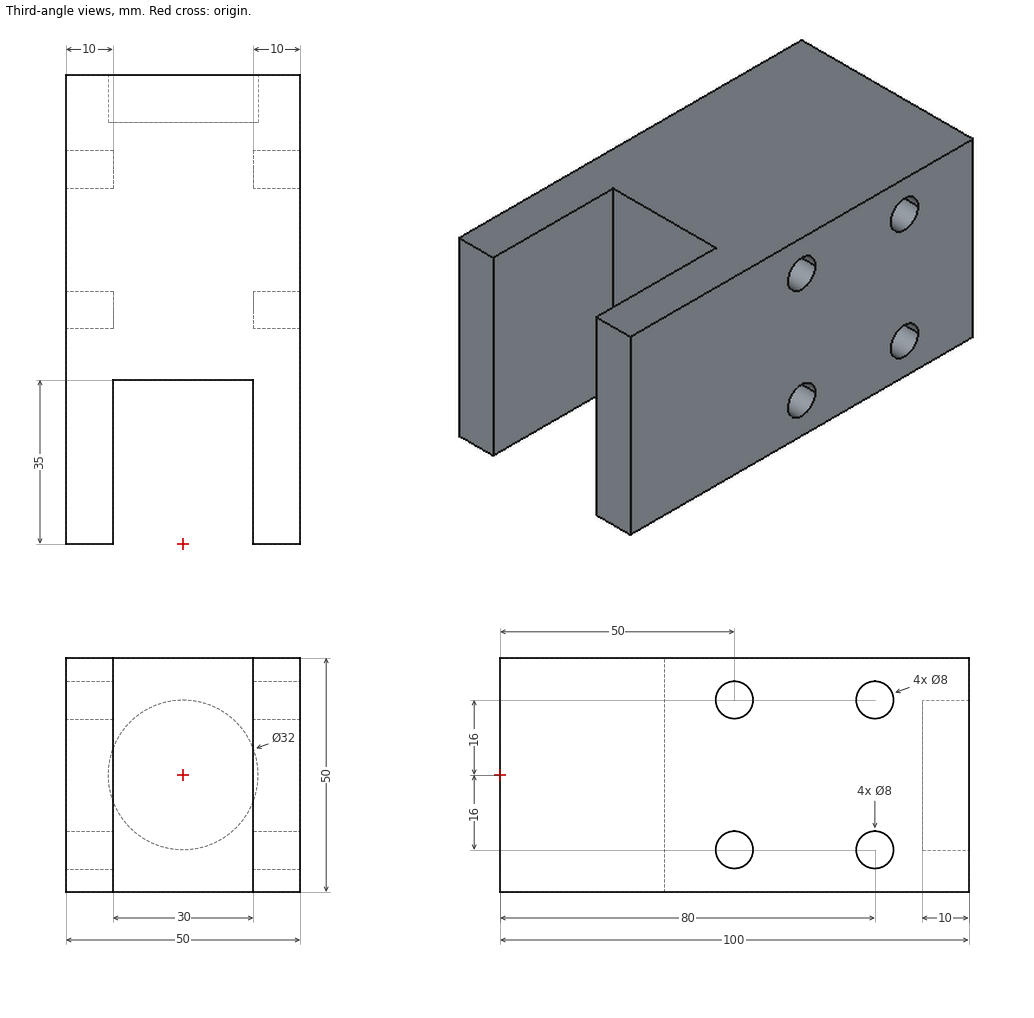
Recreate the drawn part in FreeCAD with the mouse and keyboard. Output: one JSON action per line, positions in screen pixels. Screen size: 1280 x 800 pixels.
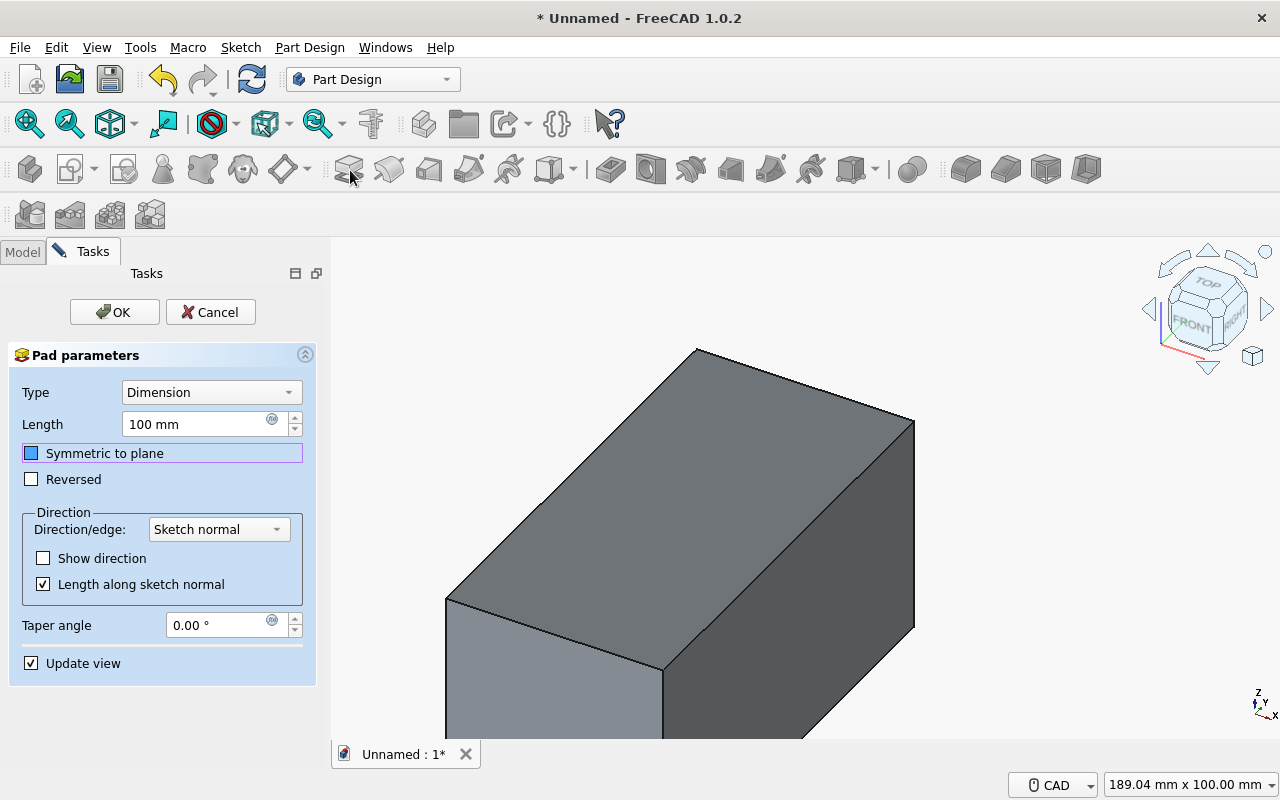
{"action": "left_click", "coordinate": [30, 479]}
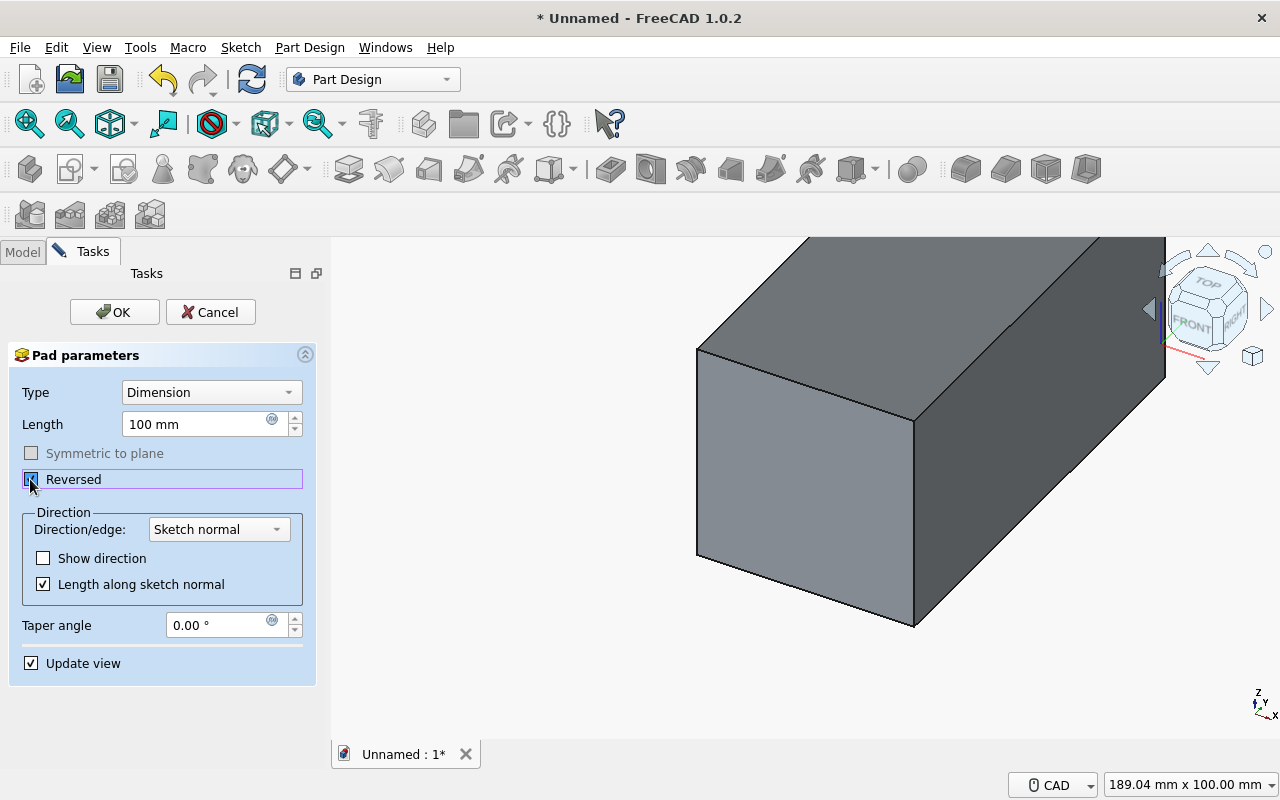
{"action": "left_click", "coordinate": [115, 312]}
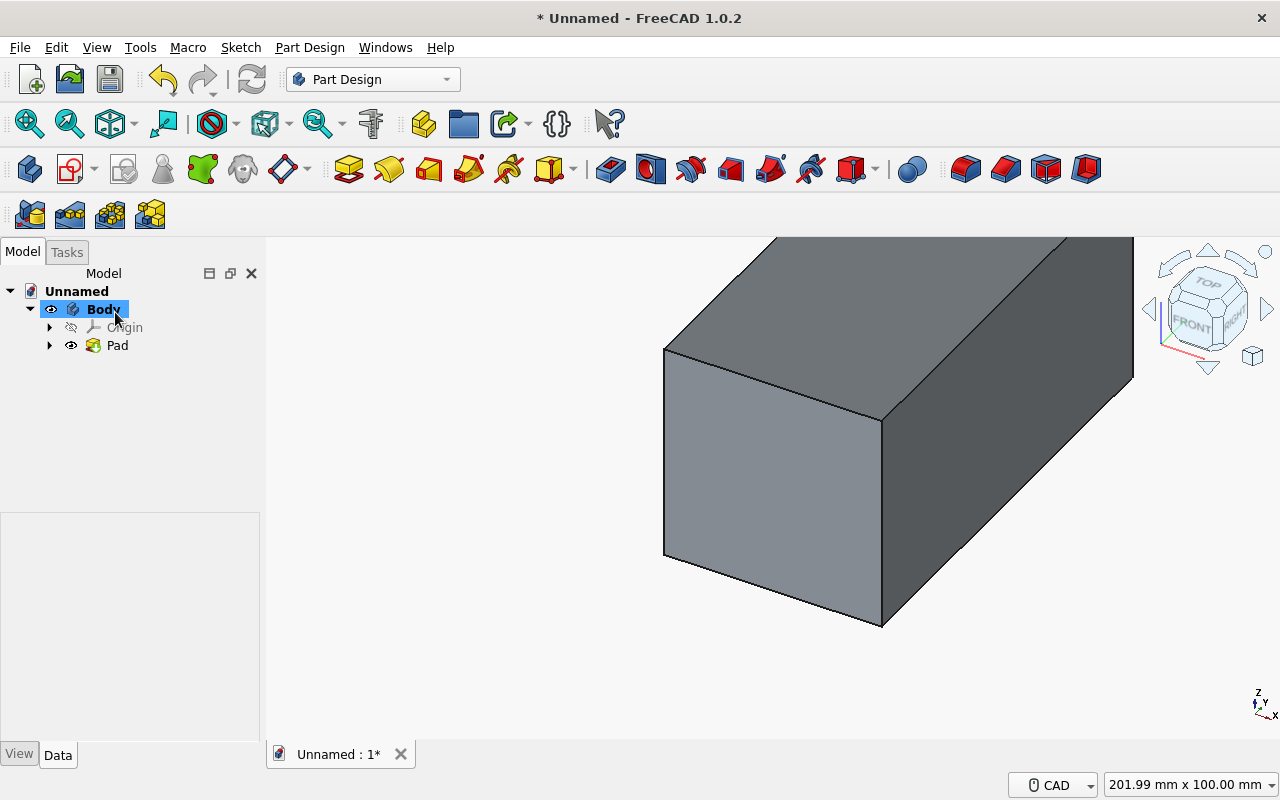
{"action": "left_click", "coordinate": [30, 124]}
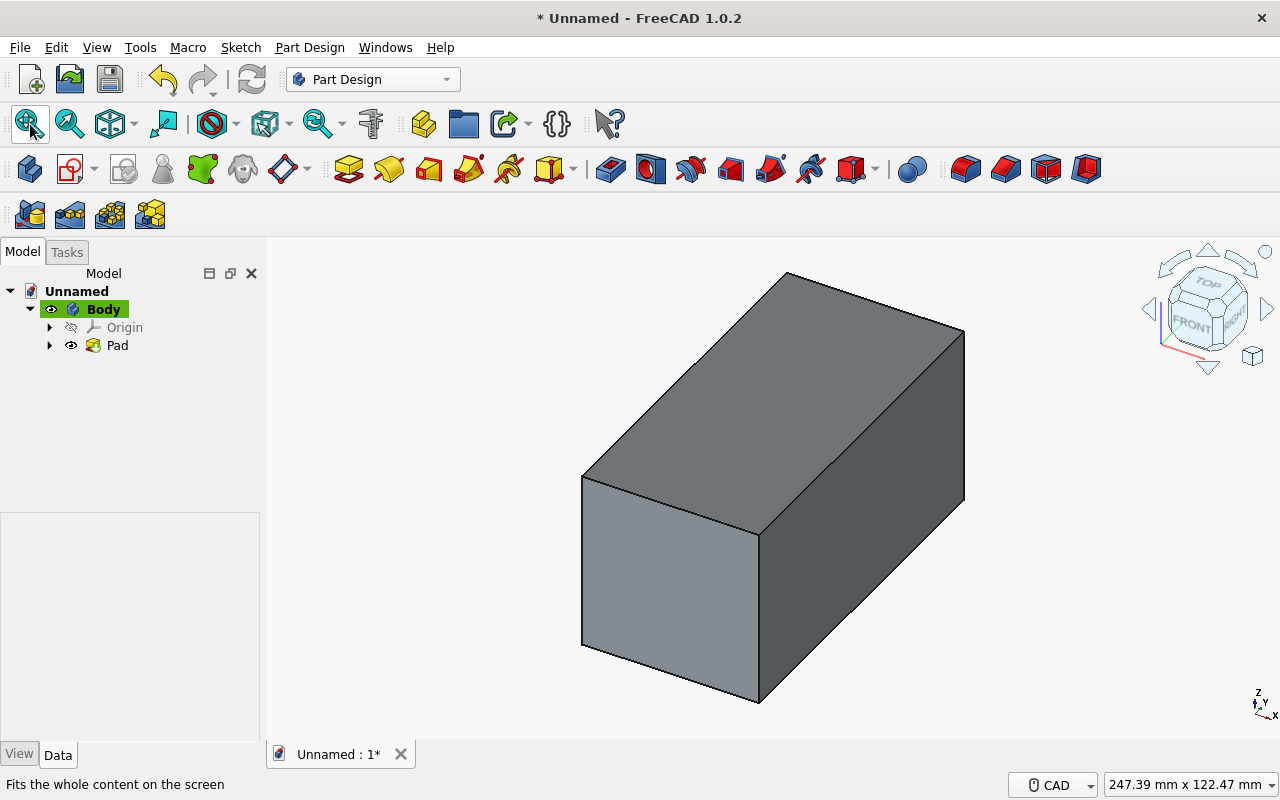
{"action": "left_click", "coordinate": [671, 589]}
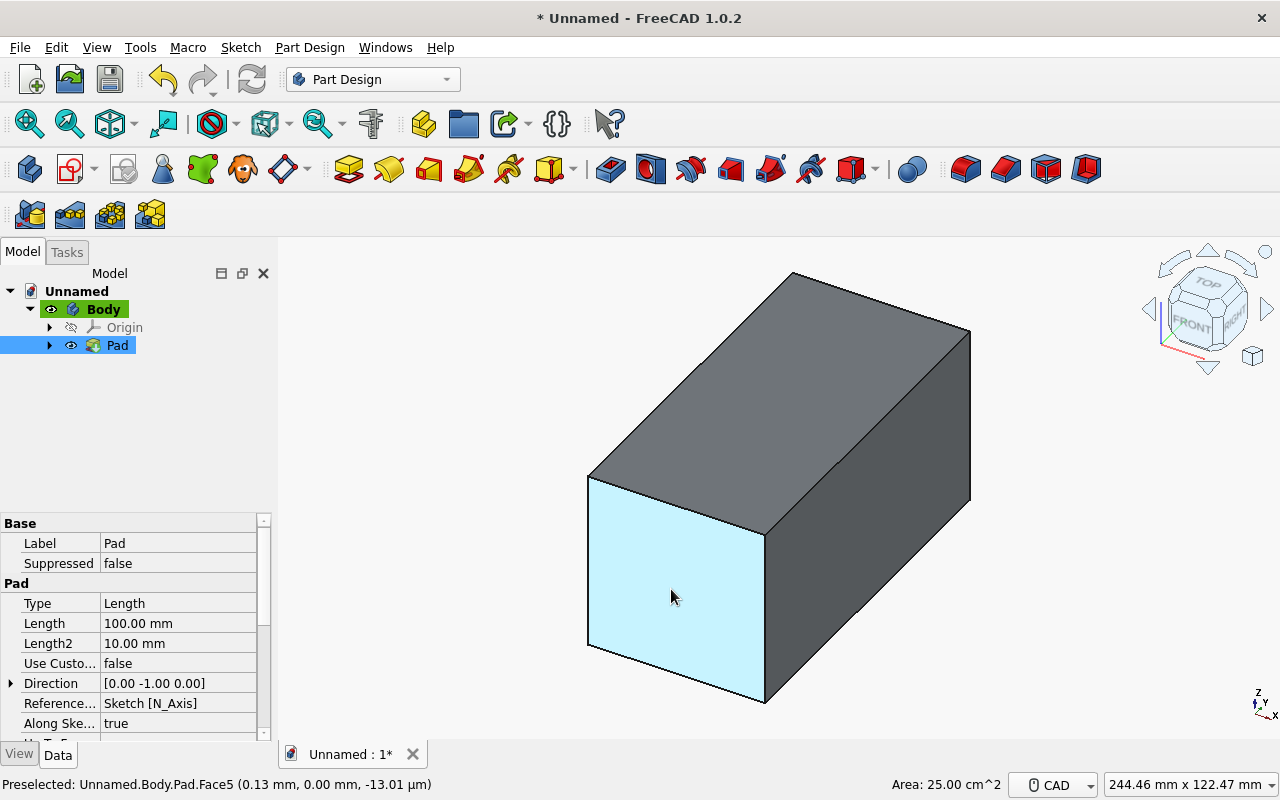
{"action": "left_click", "coordinate": [70, 170]}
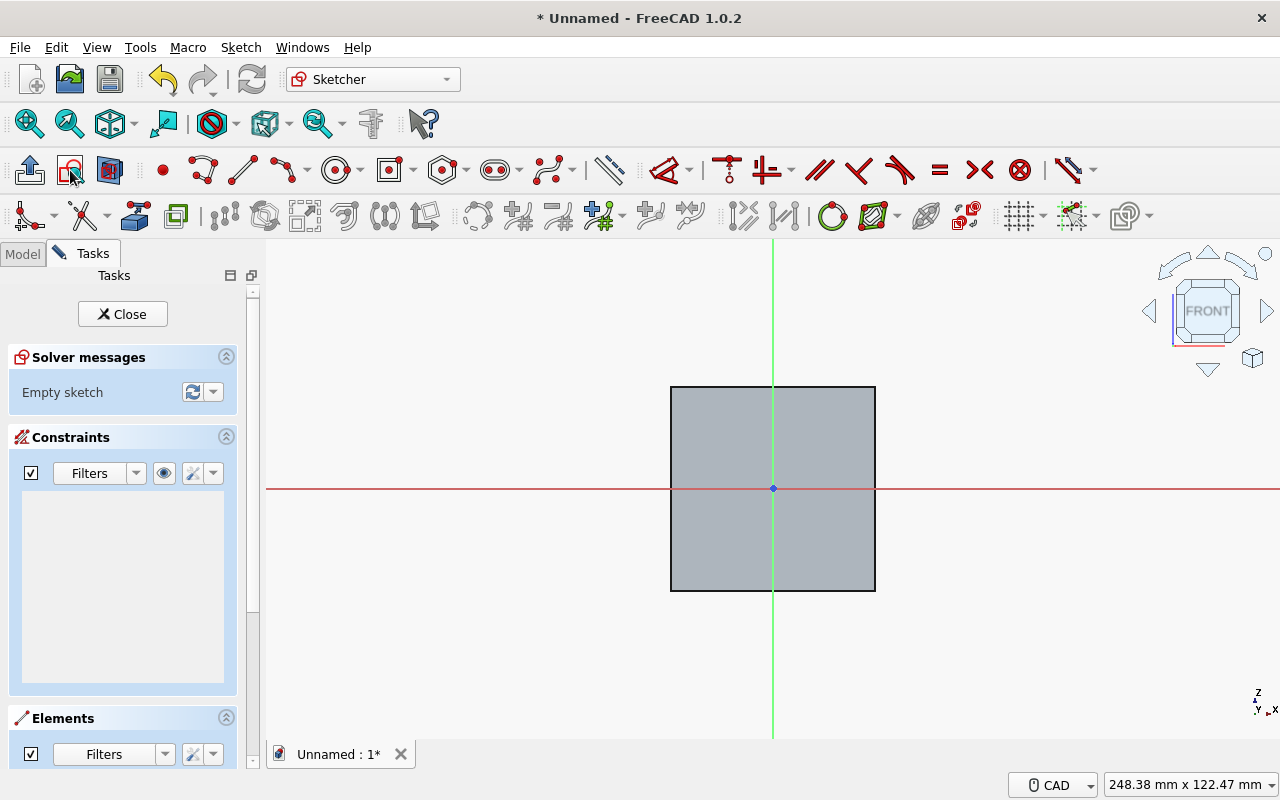
{"action": "scroll", "coordinate": [912, 489], "scroll_direction": "up", "scroll_amount": 2}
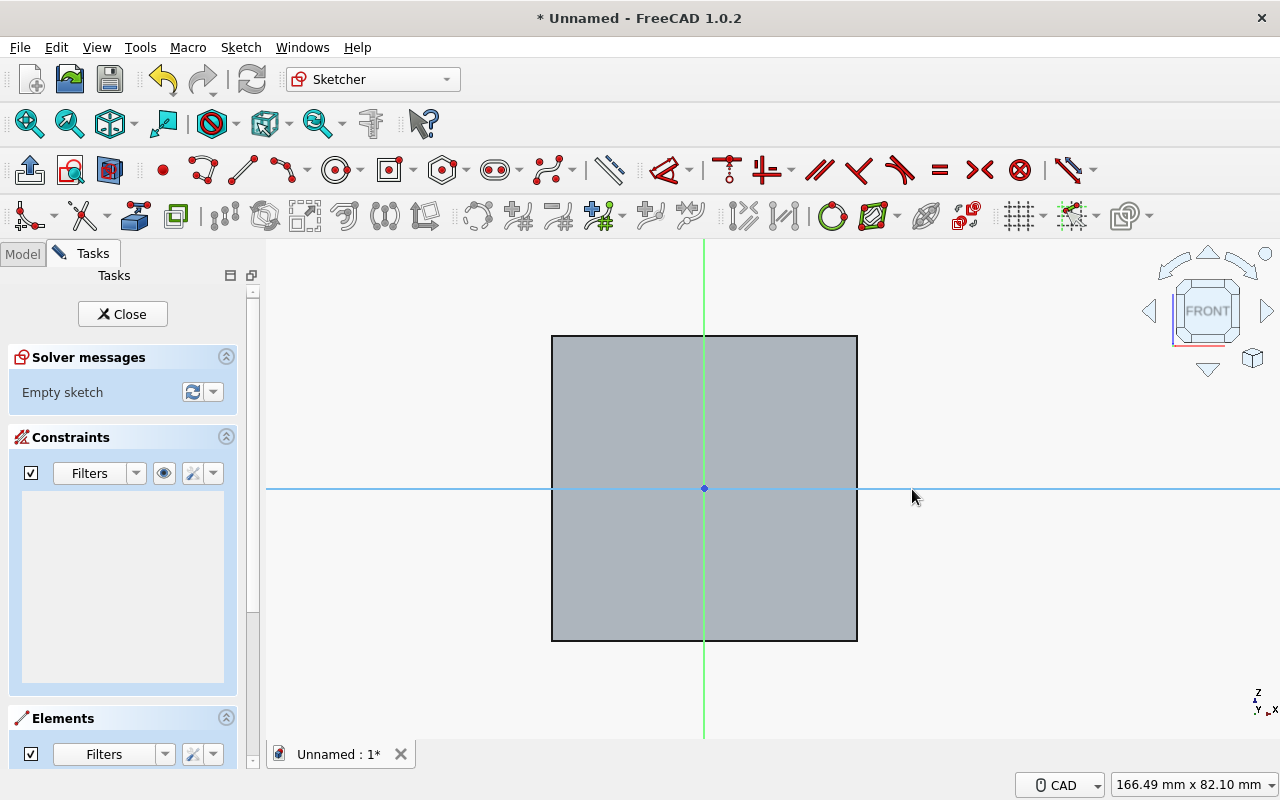
{"action": "left_click", "coordinate": [390, 170]}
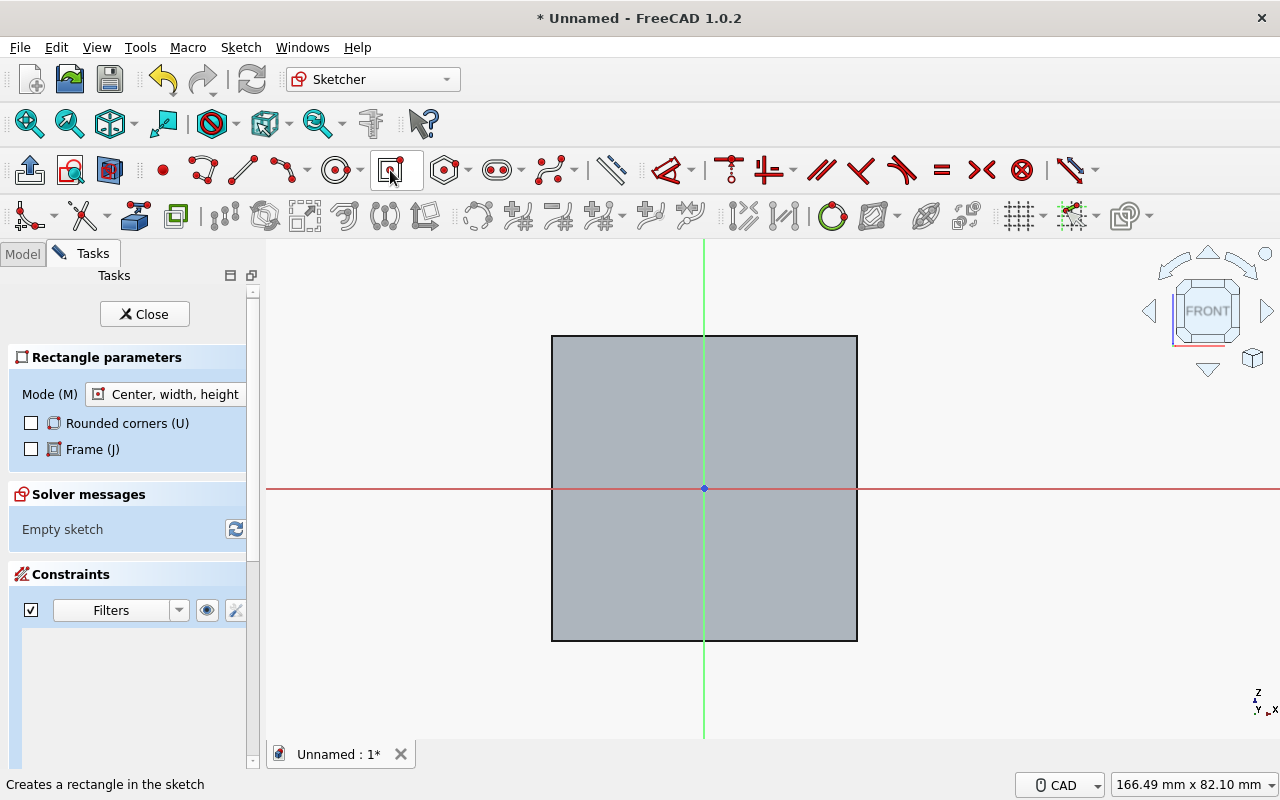
{"action": "left_click", "coordinate": [704, 489]}
{"action": "mouse_move", "coordinate": [796, 336]}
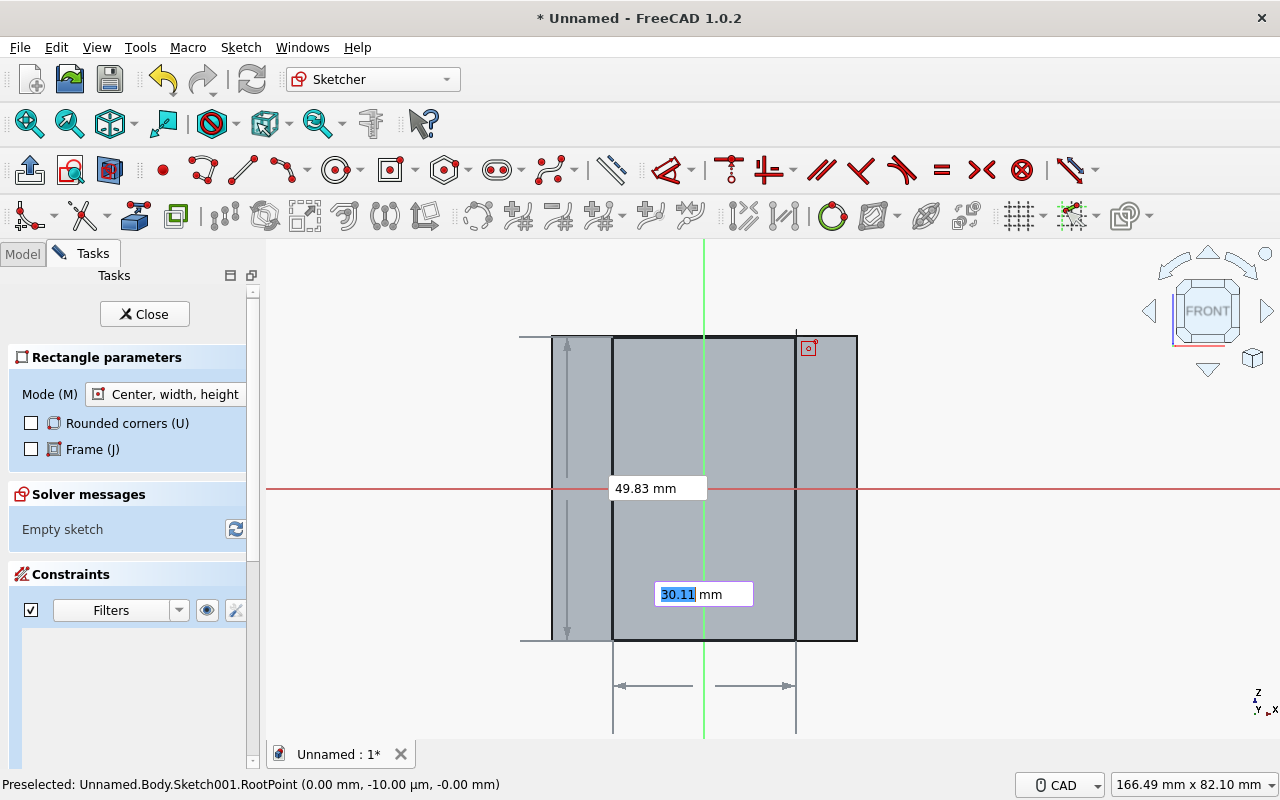
{"action": "type", "text": "30"}
{"action": "key", "text": "Tab"}
{"action": "type", "text": "50"}
{"action": "key", "text": "Return"}
{"action": "key", "text": "Escape"}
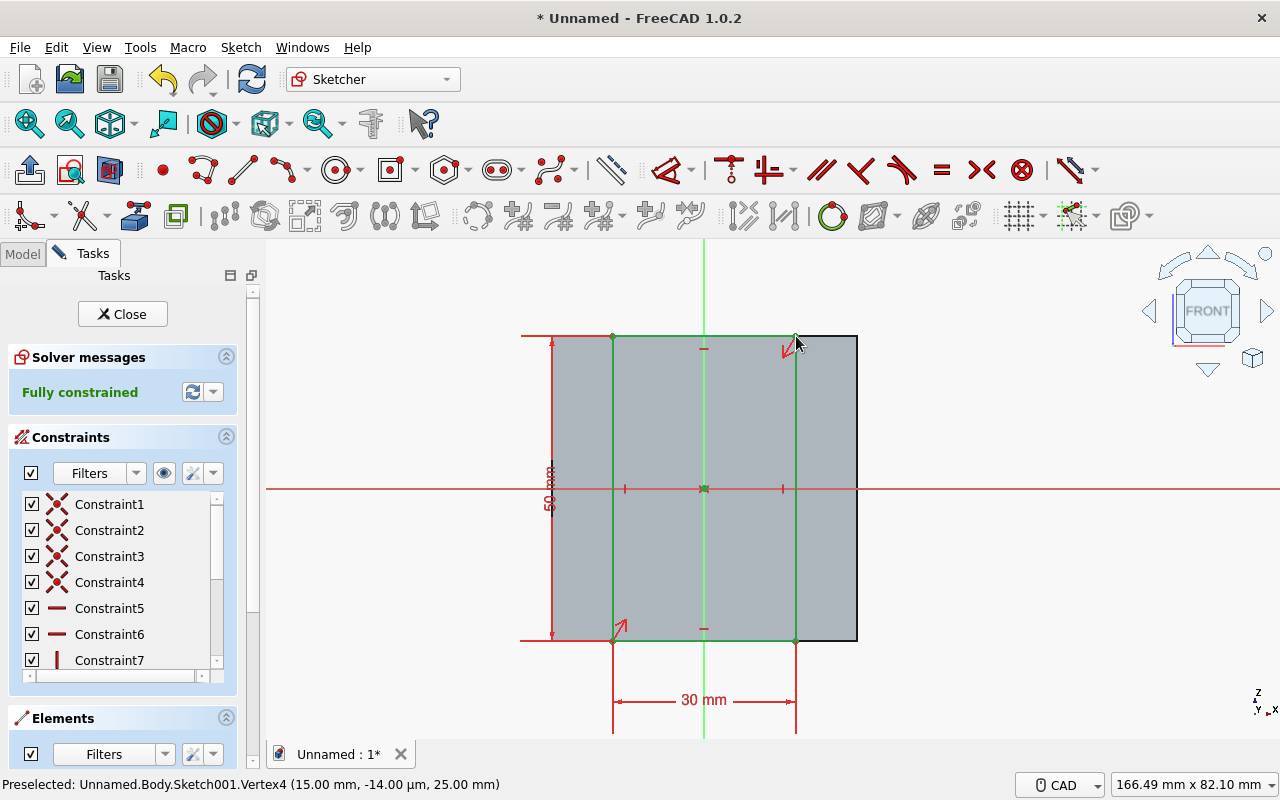
{"action": "left_click", "coordinate": [123, 314]}